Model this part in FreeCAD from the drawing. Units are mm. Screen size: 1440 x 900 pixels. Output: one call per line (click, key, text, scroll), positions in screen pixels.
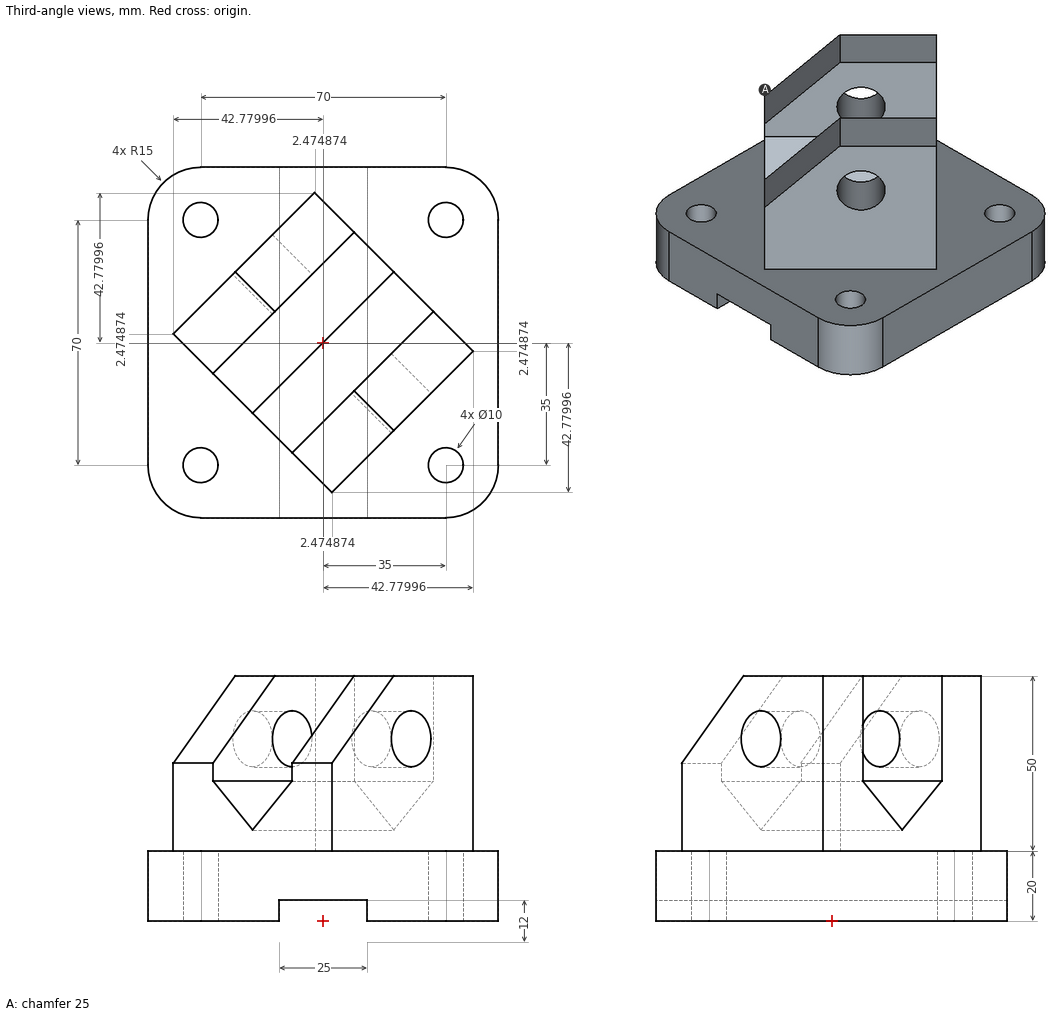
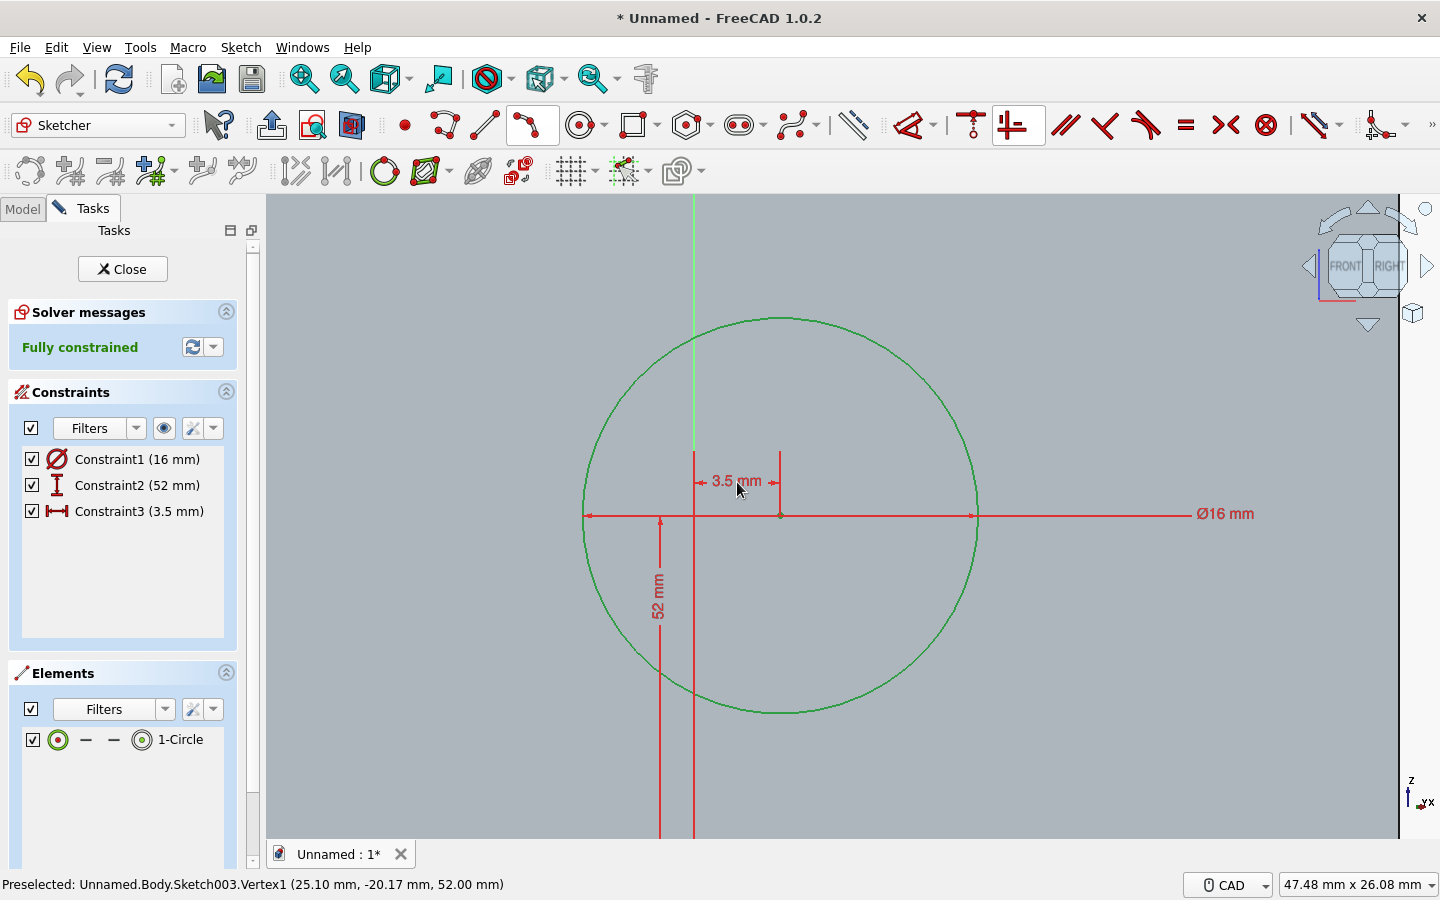
click(123, 269)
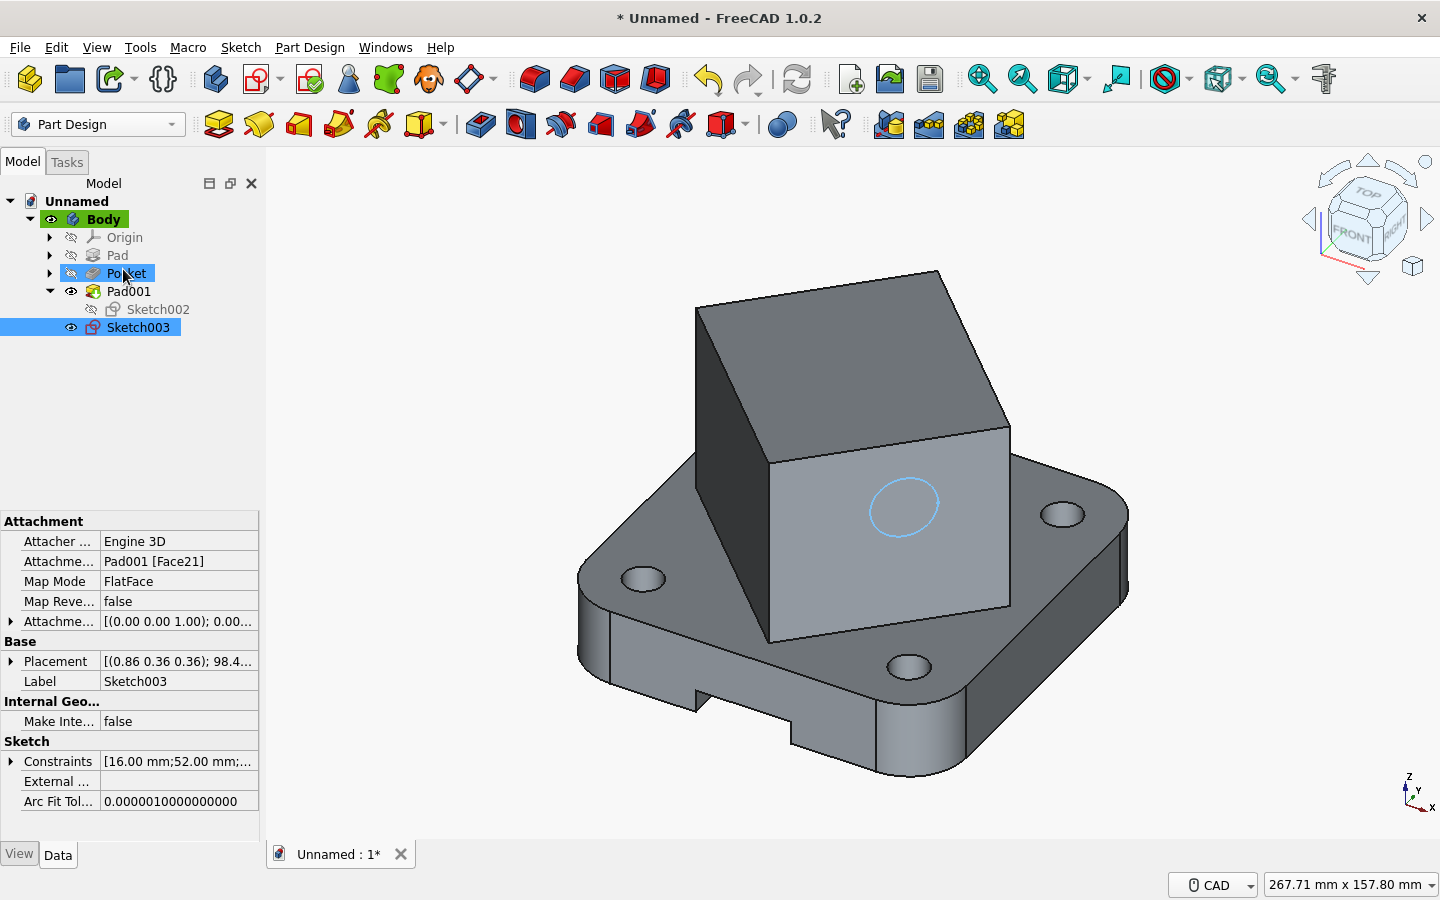
click(482, 124)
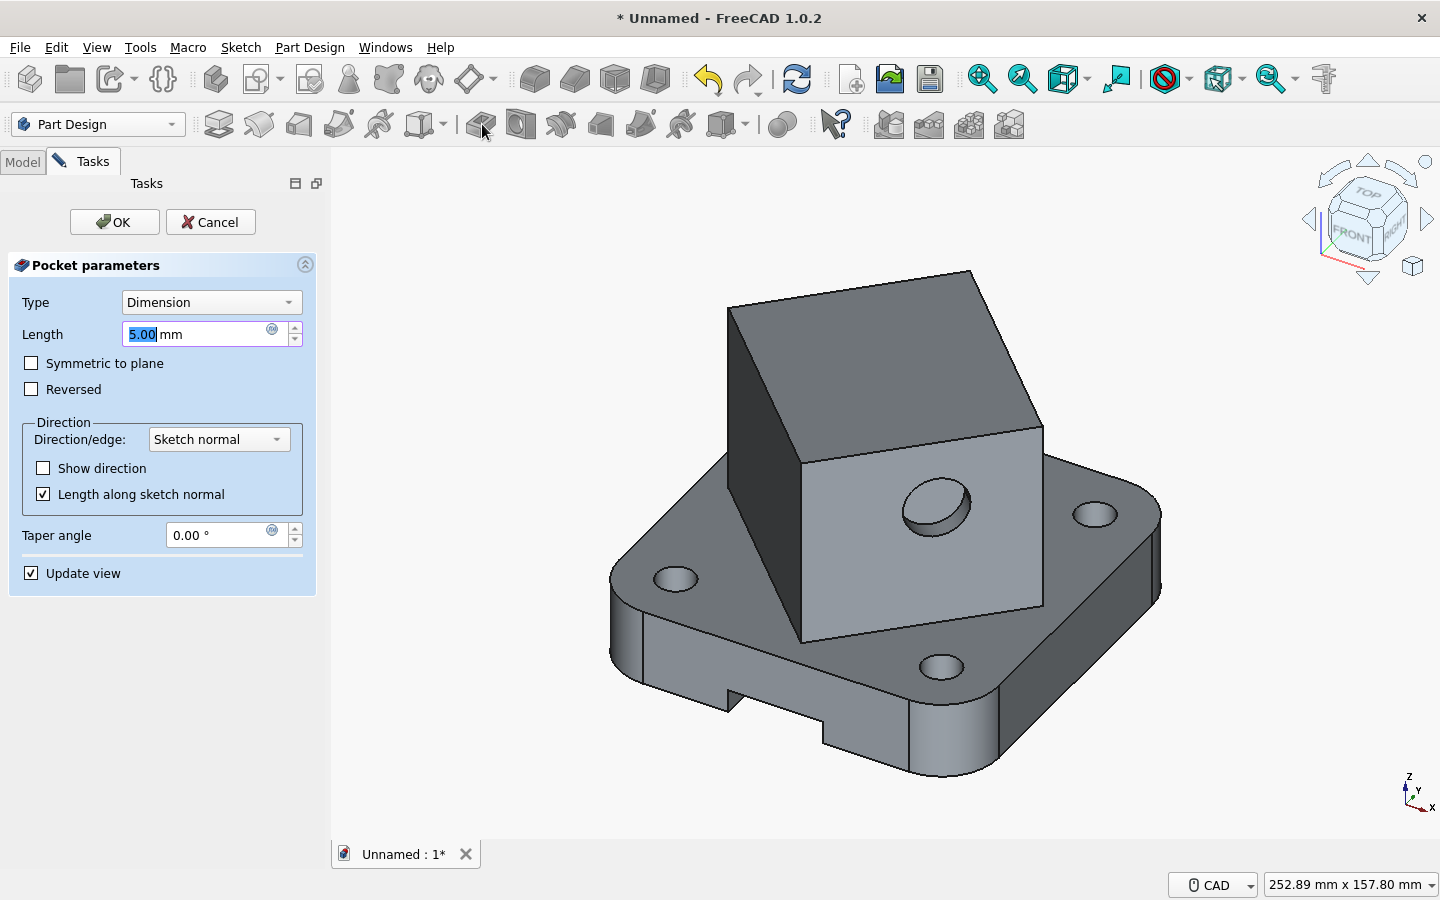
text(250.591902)
key(Tab)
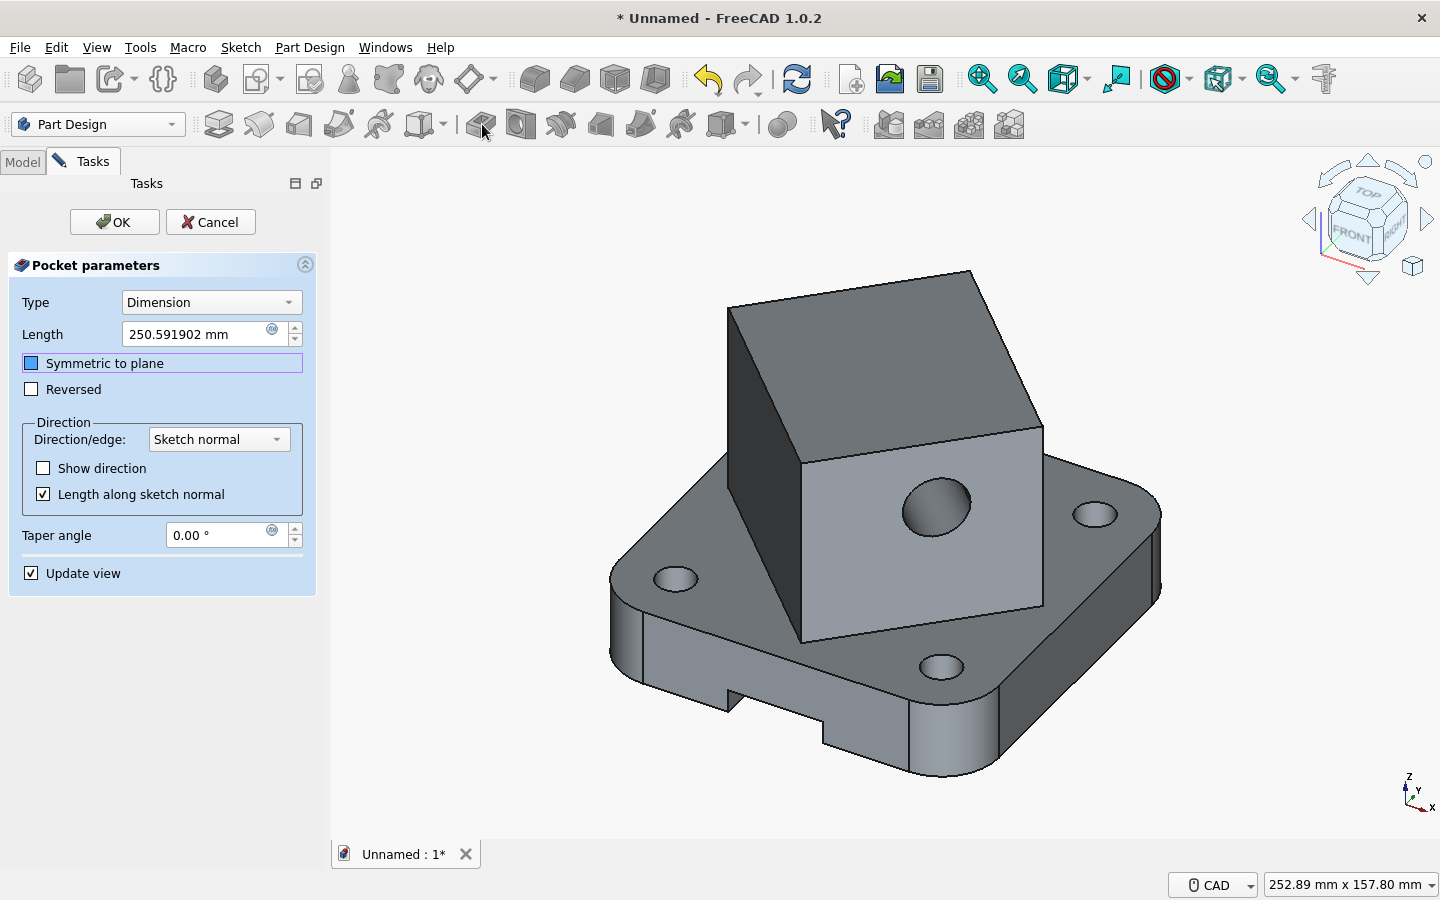
click(30, 363)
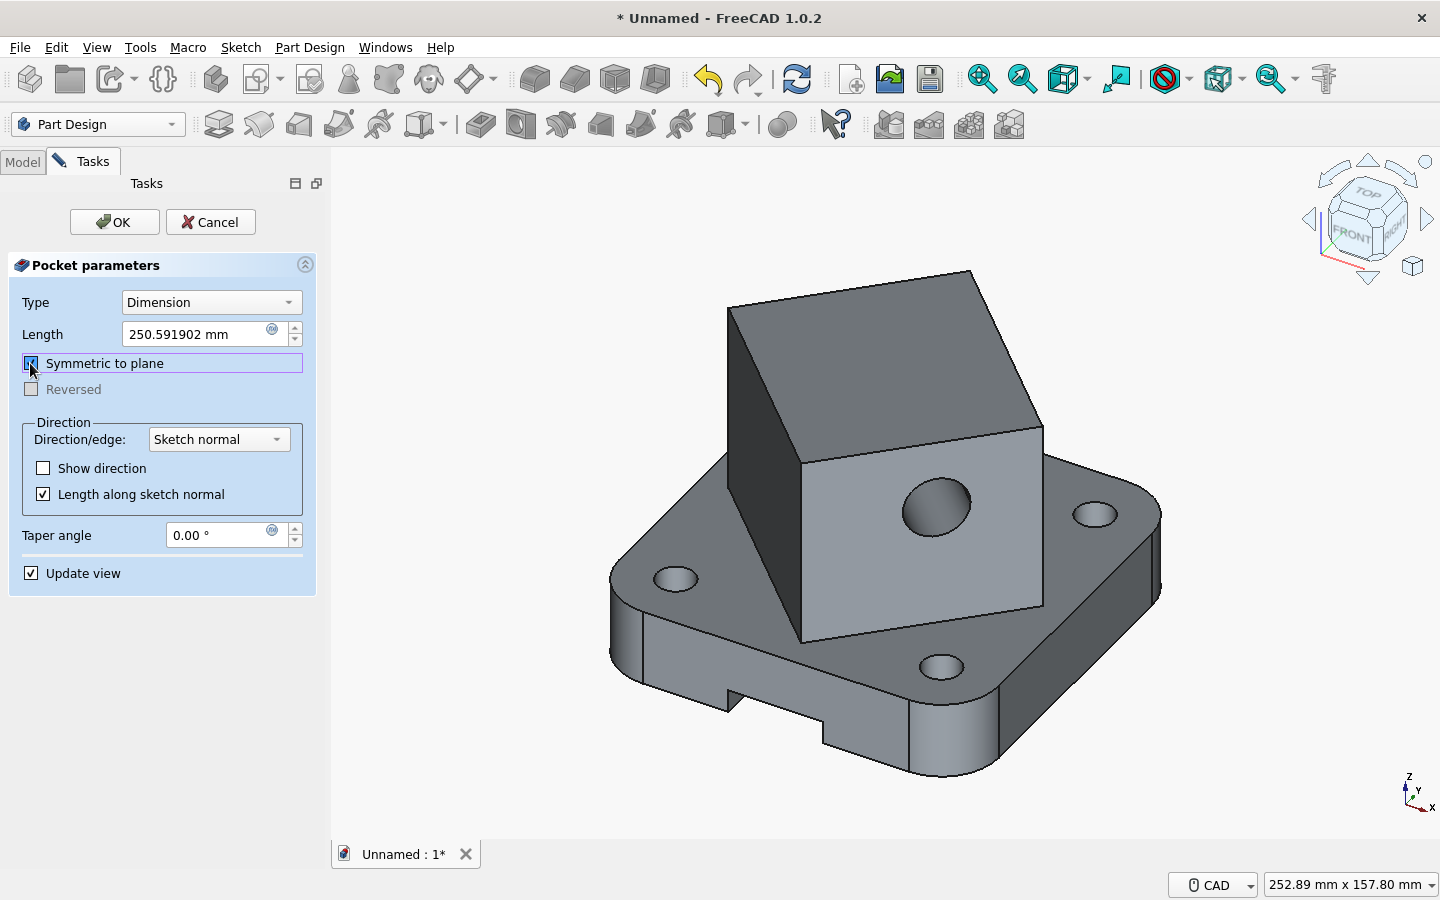
click(115, 222)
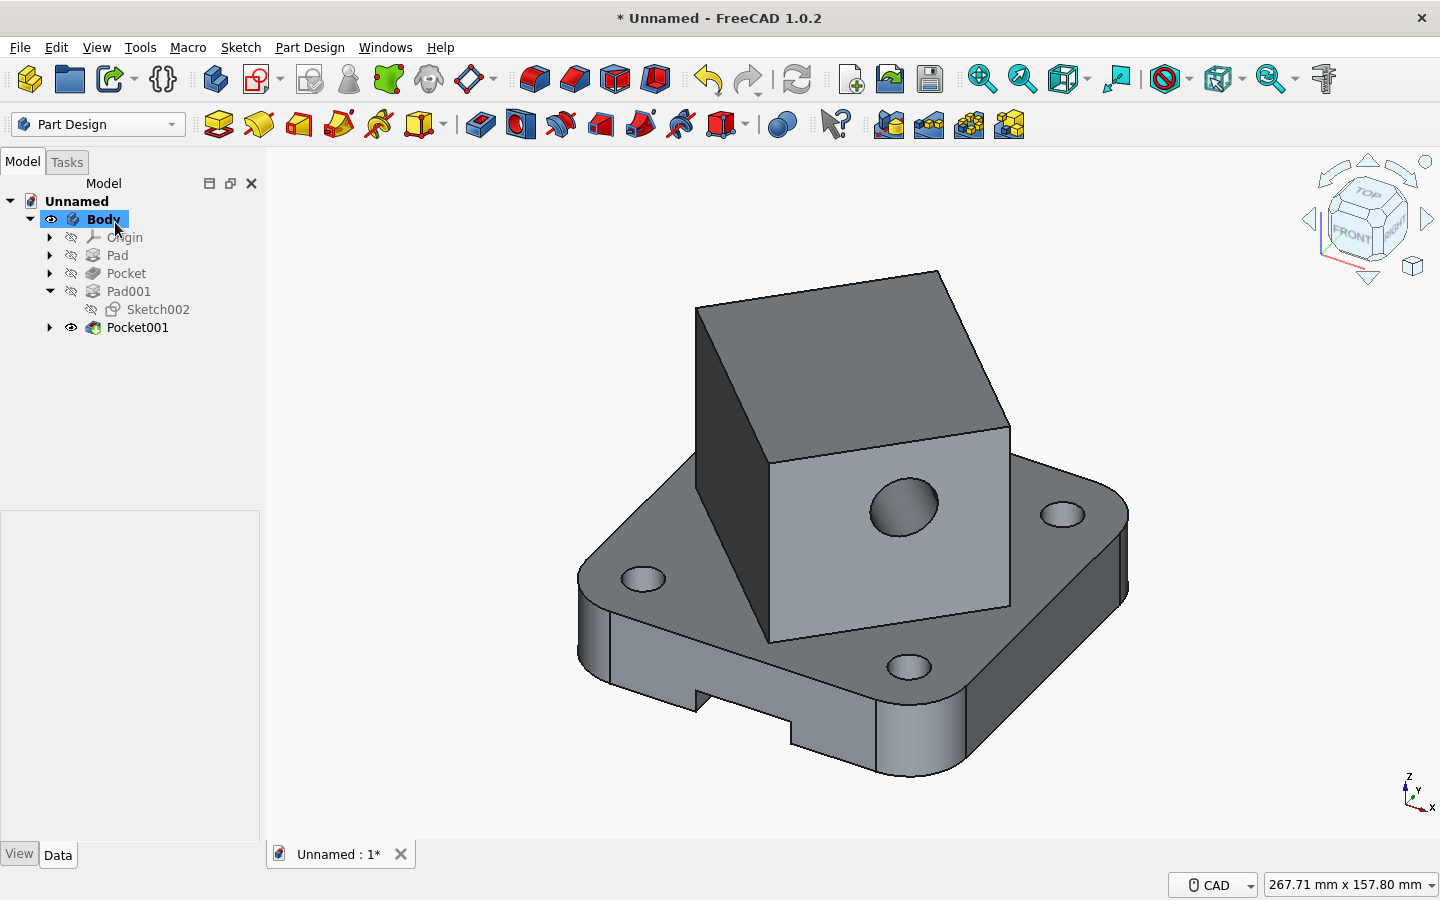
click(732, 385)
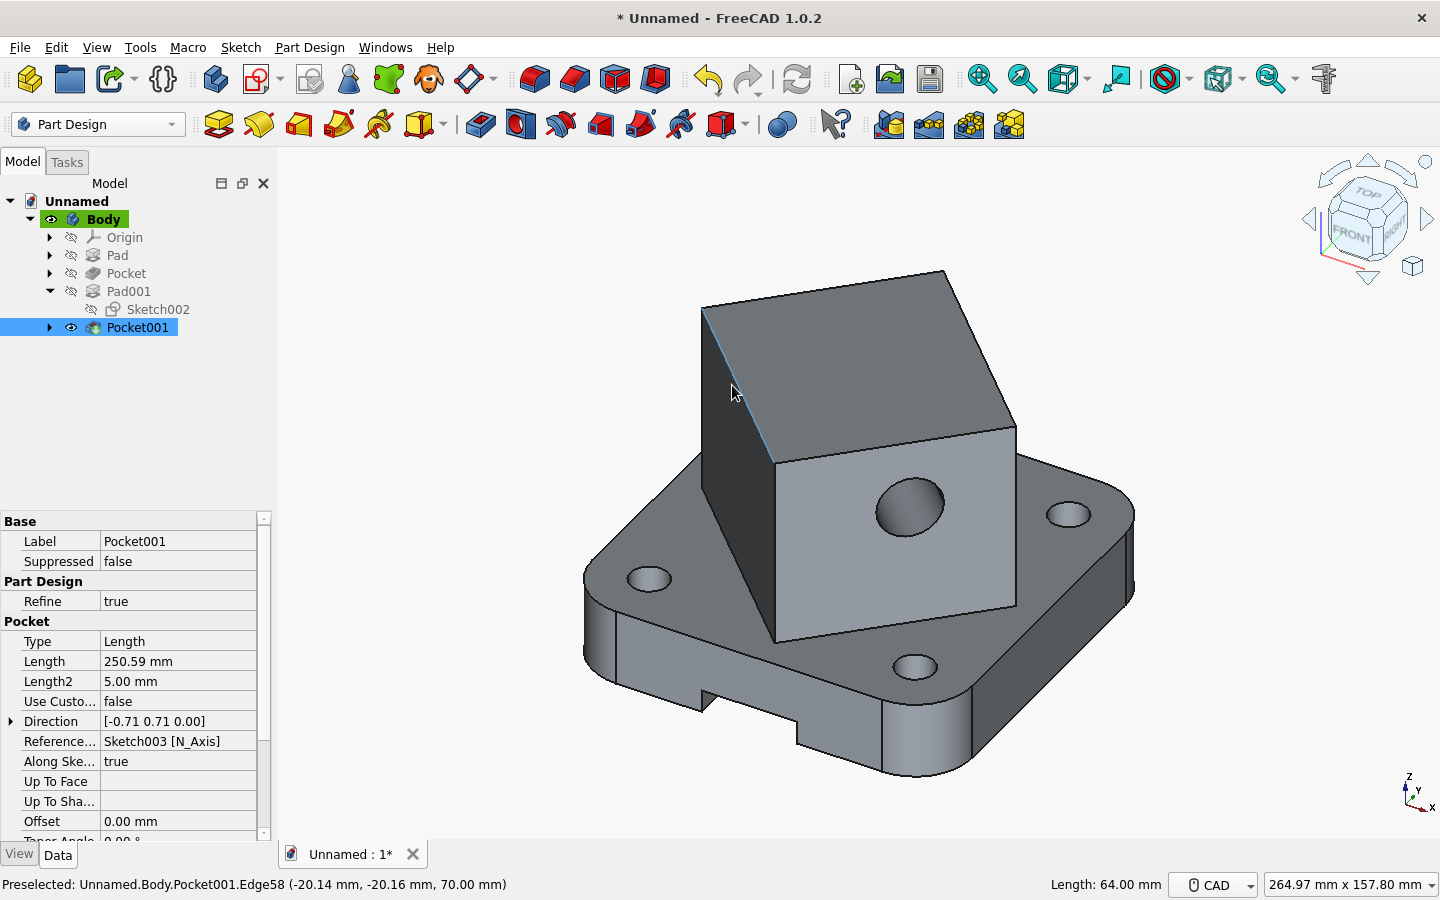
click(576, 80)